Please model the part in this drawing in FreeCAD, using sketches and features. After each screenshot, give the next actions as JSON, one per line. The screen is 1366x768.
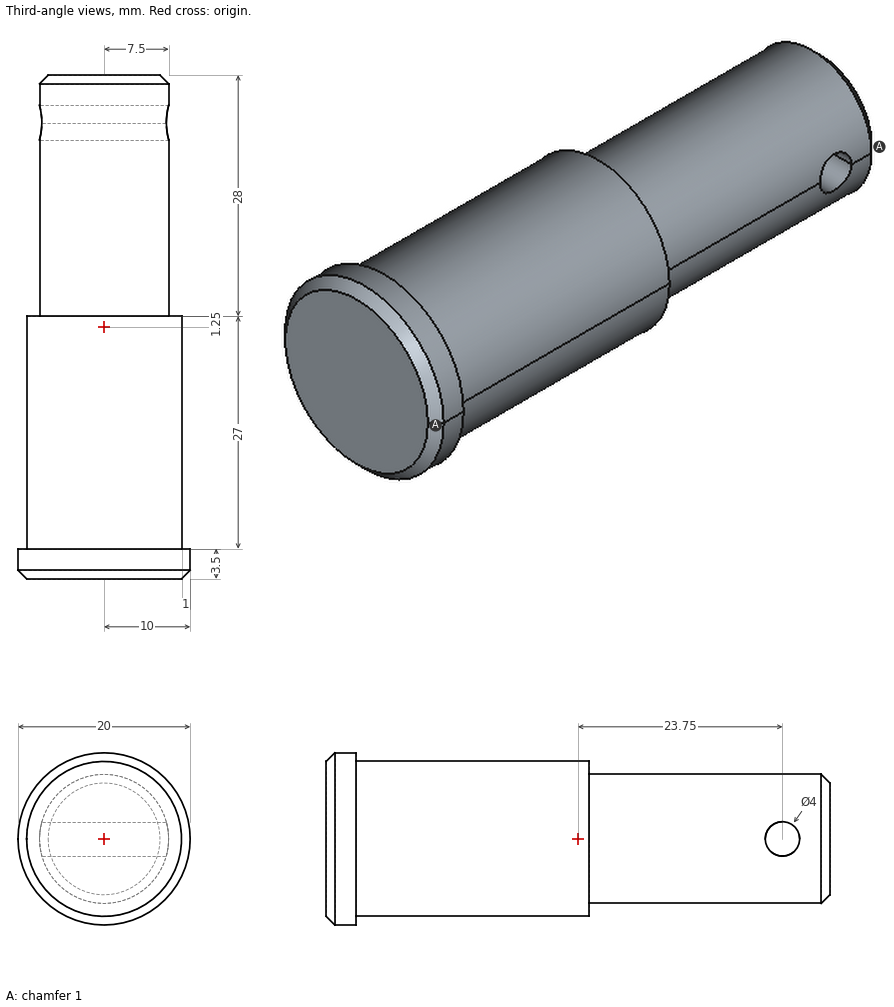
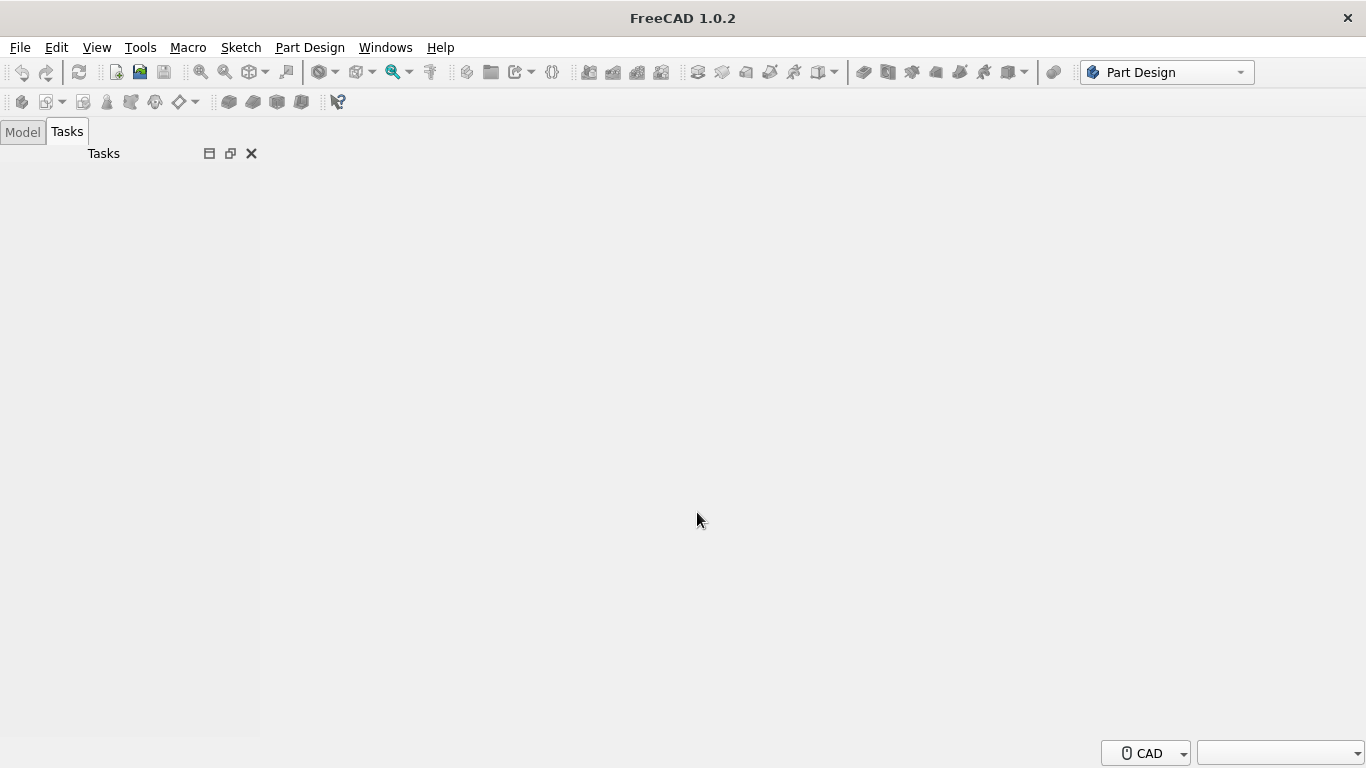
{"action": "left_click", "coordinate": [116, 72]}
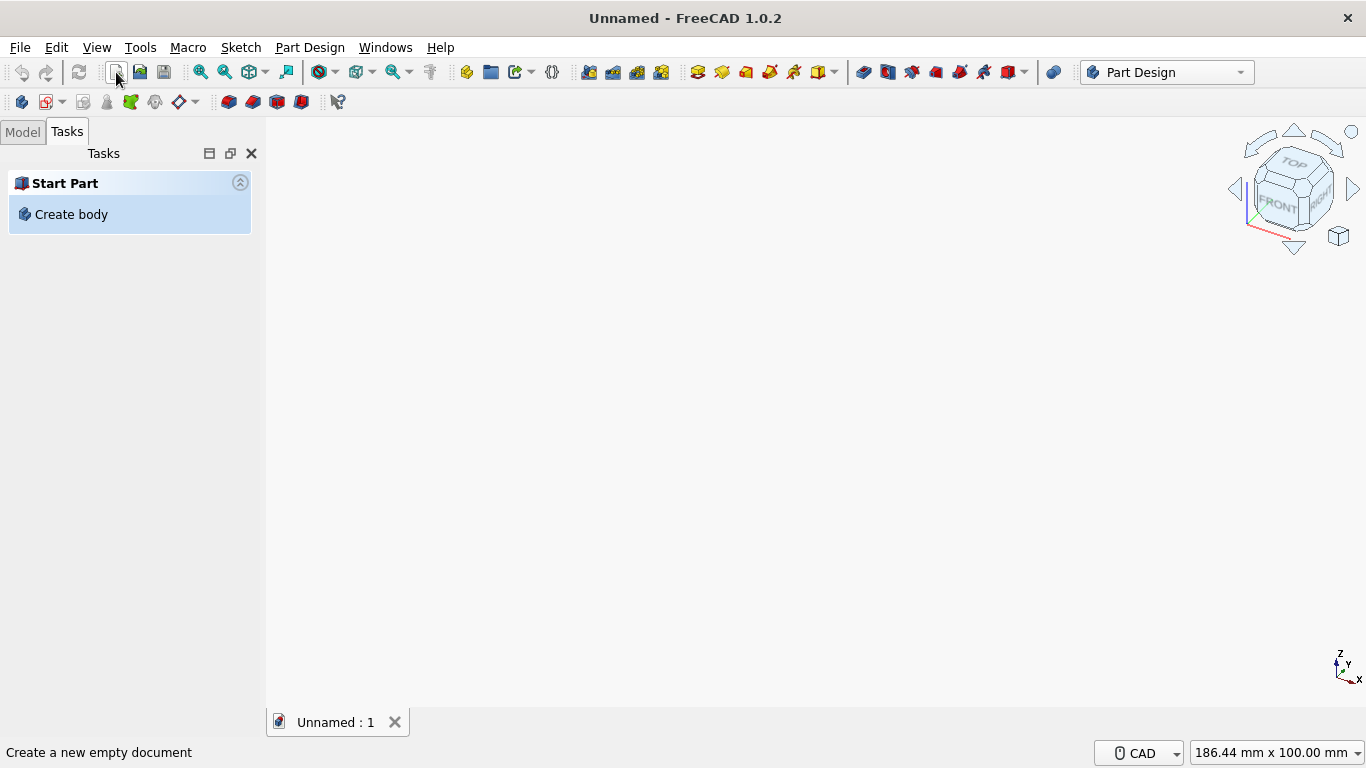
{"action": "left_click", "coordinate": [46, 102]}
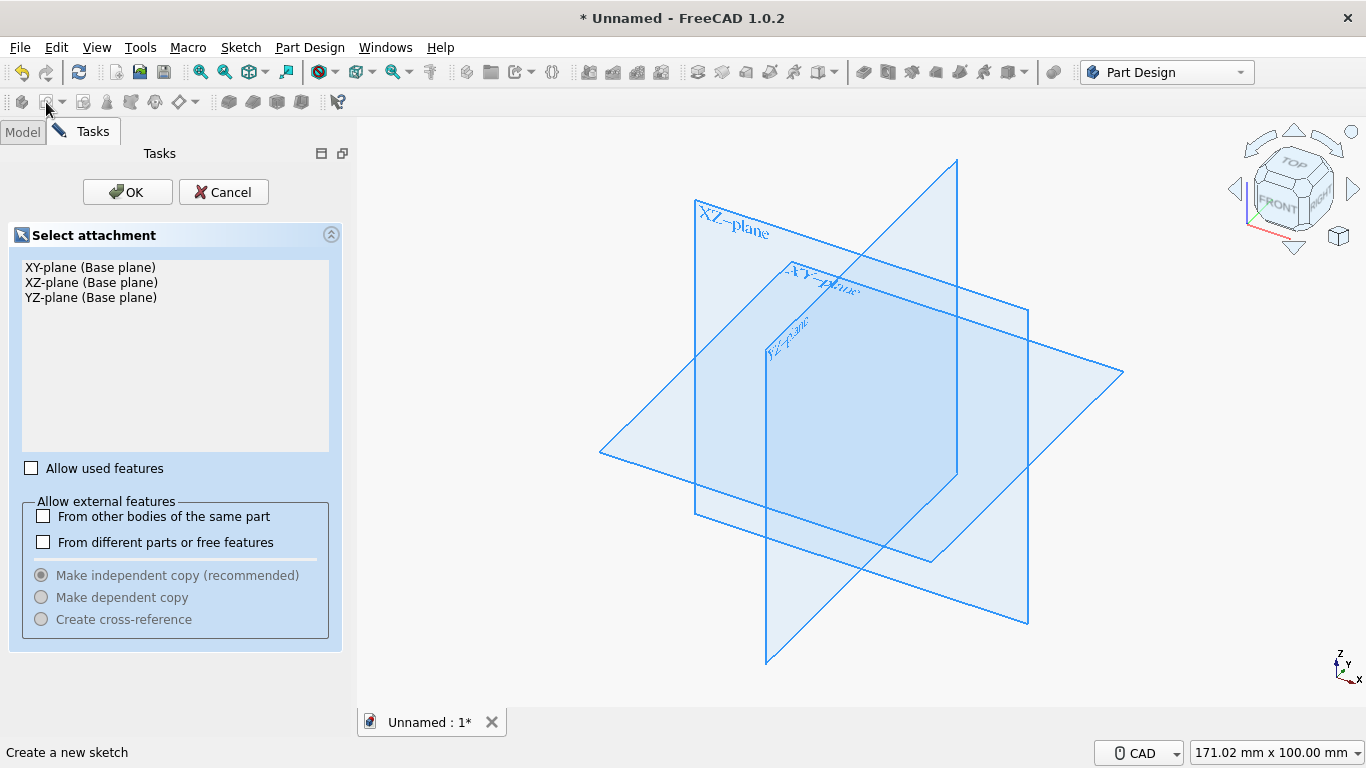
{"action": "left_click", "coordinate": [82, 268]}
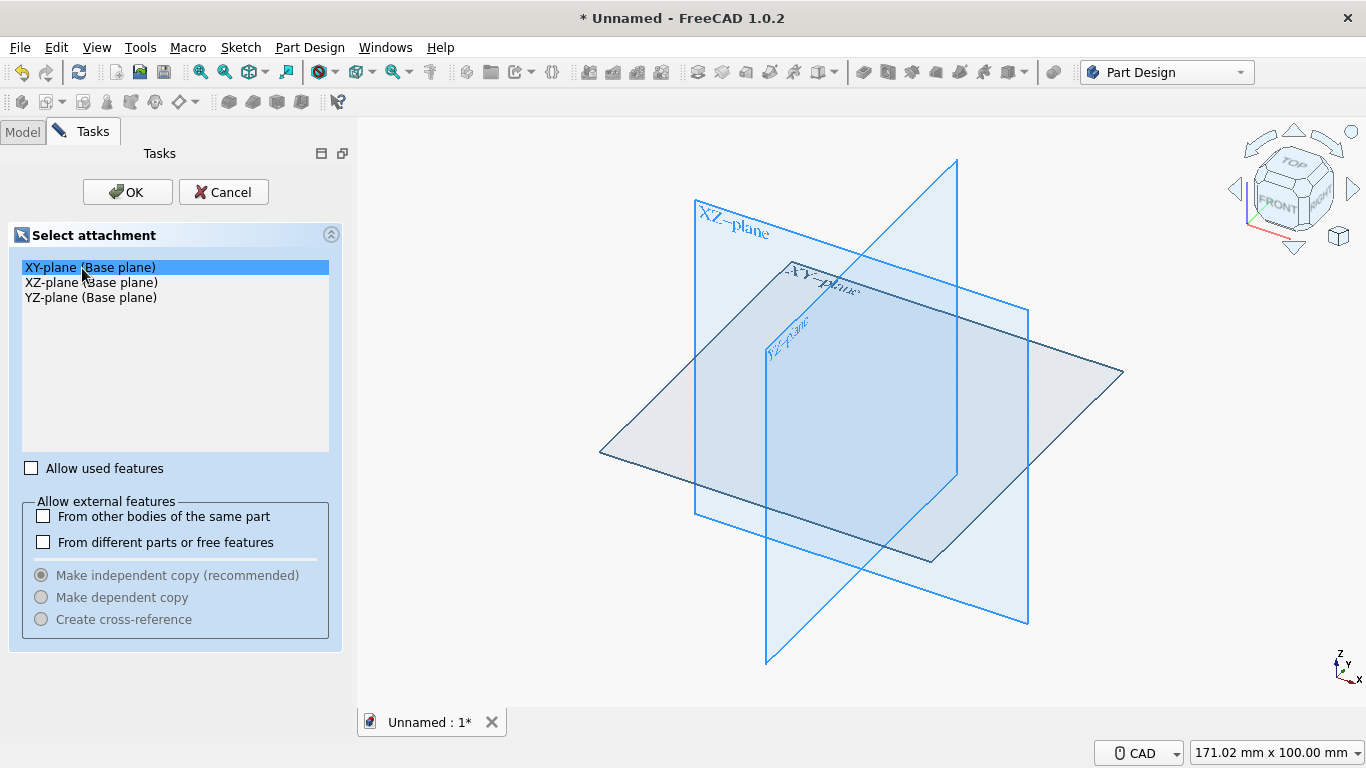
{"action": "left_click", "coordinate": [128, 192]}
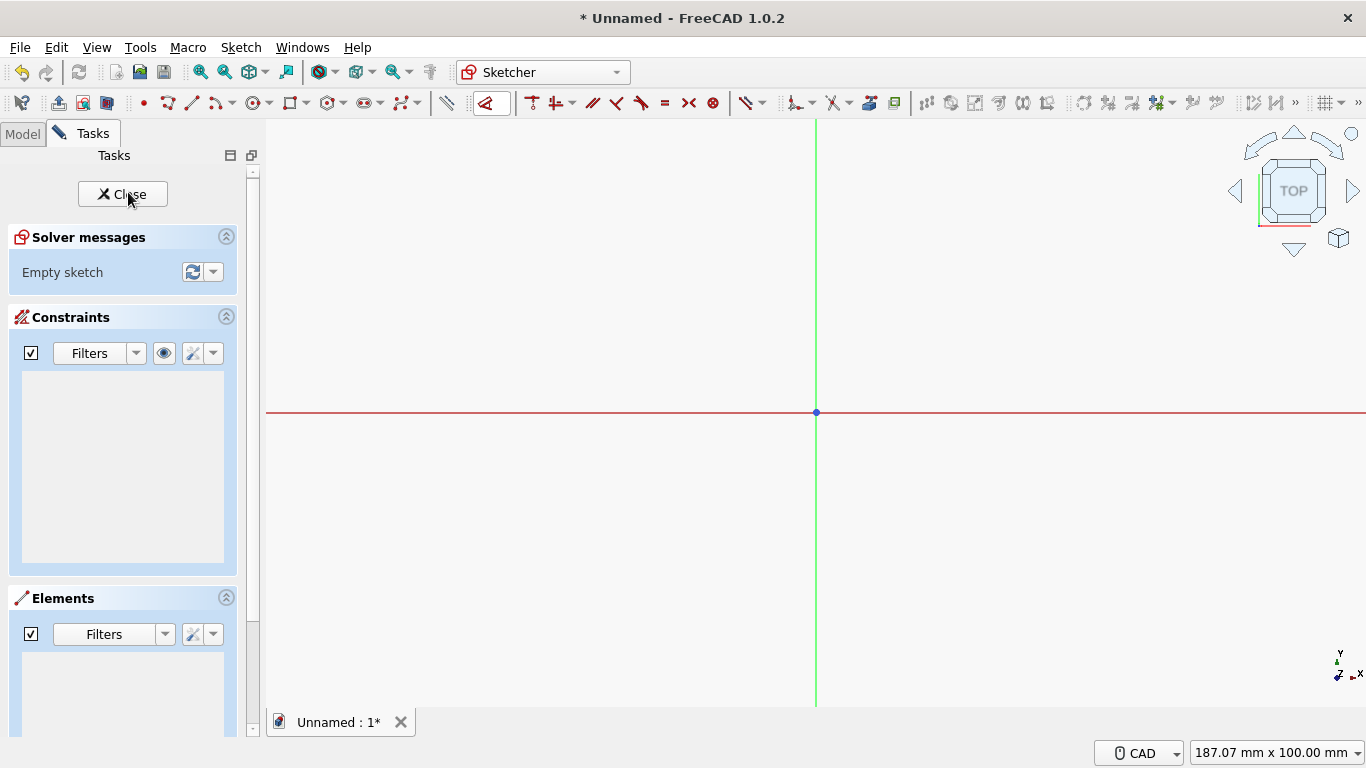
{"action": "left_click", "coordinate": [168, 104]}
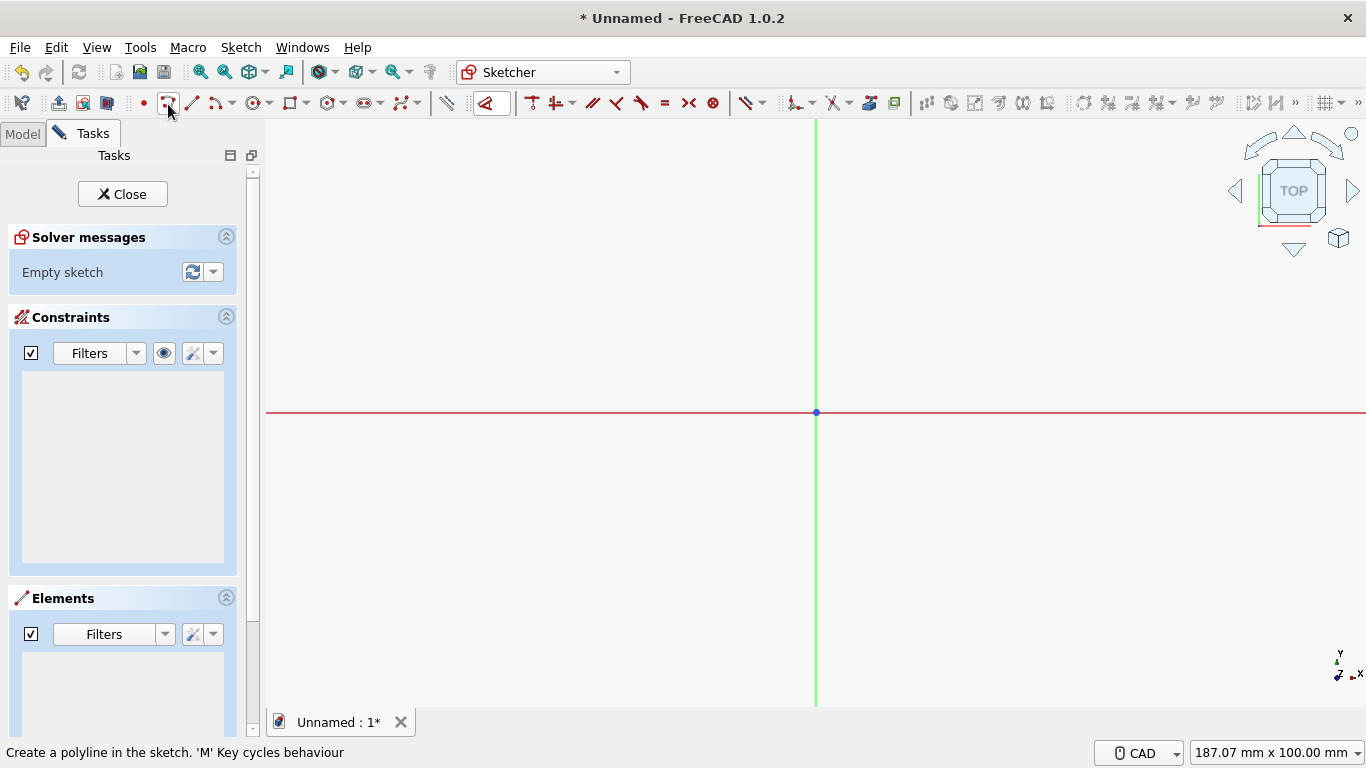
{"action": "scroll", "coordinate": [860, 406], "scroll_direction": "up", "scroll_amount": 4}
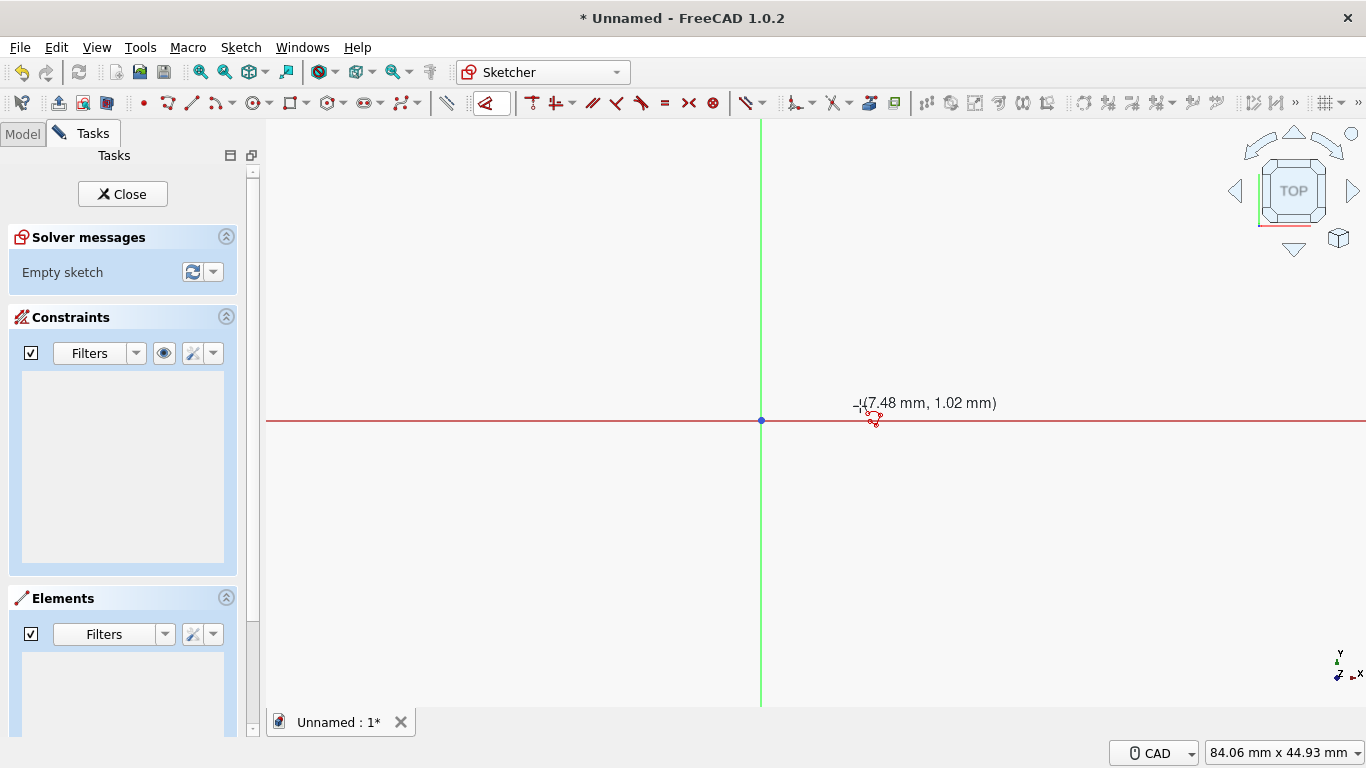
{"action": "left_click", "coordinate": [860, 405]}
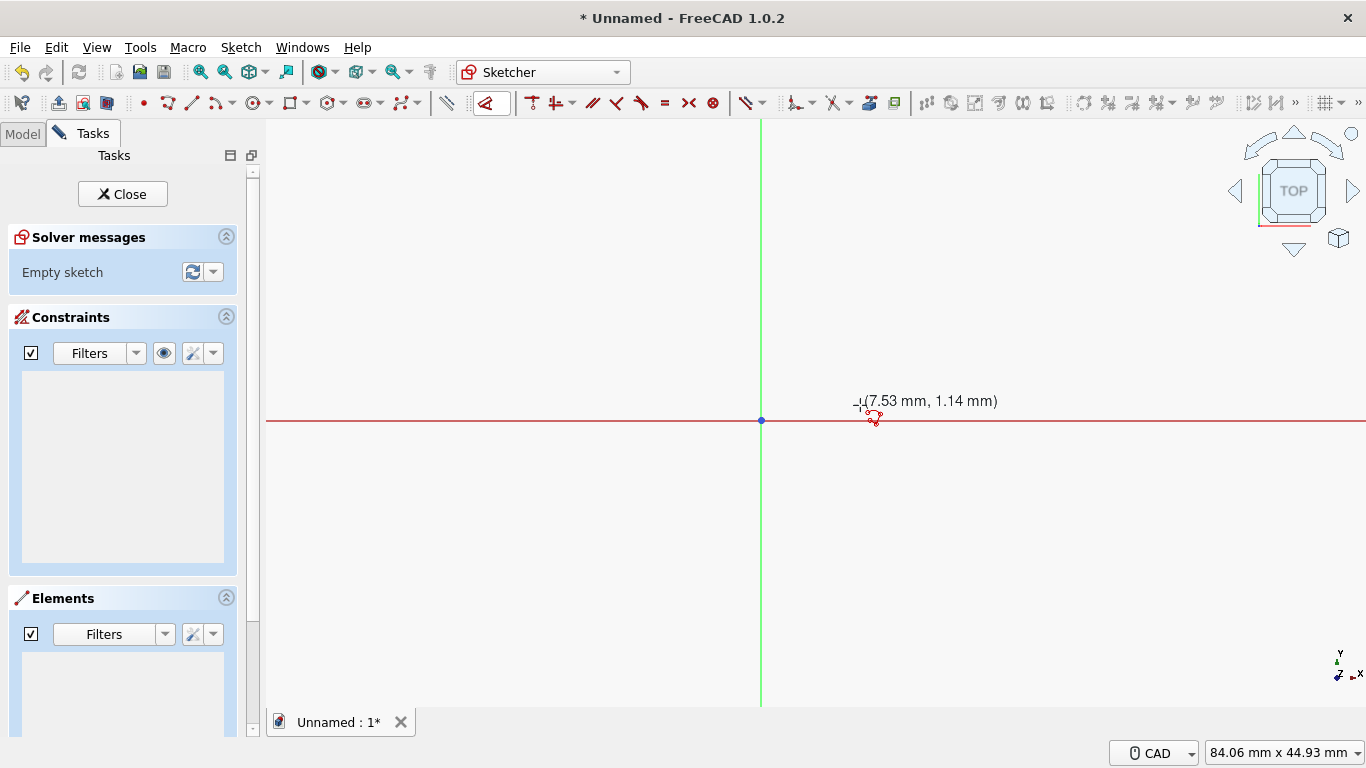
{"action": "scroll", "coordinate": [683, 406], "scroll_direction": "down", "scroll_amount": 4}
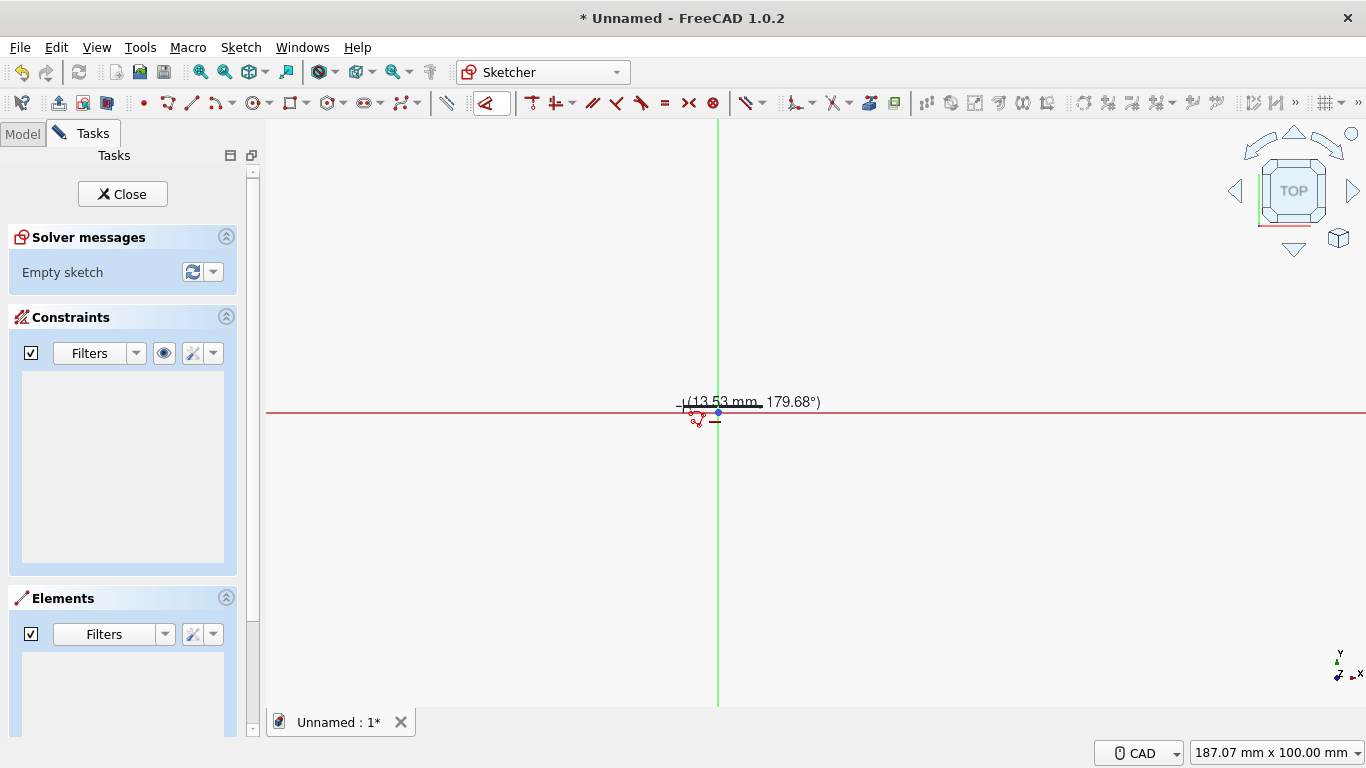
{"action": "left_click", "coordinate": [763, 241]}
{"action": "left_click", "coordinate": [718, 241]}
{"action": "left_click", "coordinate": [727, 585]}
{"action": "left_click", "coordinate": [777, 585]}
{"action": "left_click", "coordinate": [777, 564]}